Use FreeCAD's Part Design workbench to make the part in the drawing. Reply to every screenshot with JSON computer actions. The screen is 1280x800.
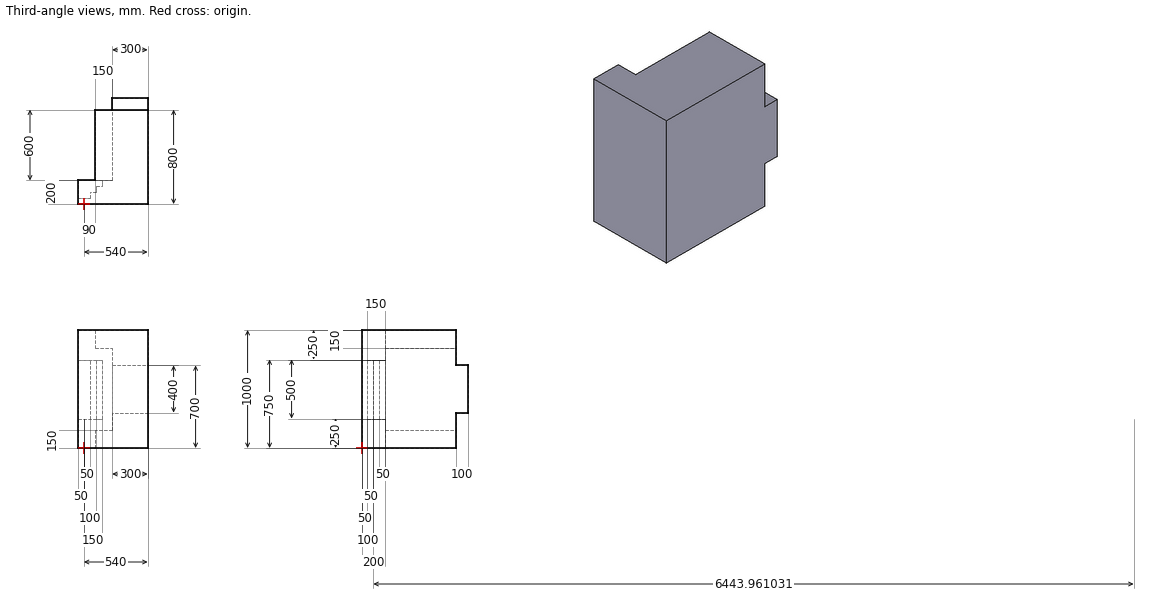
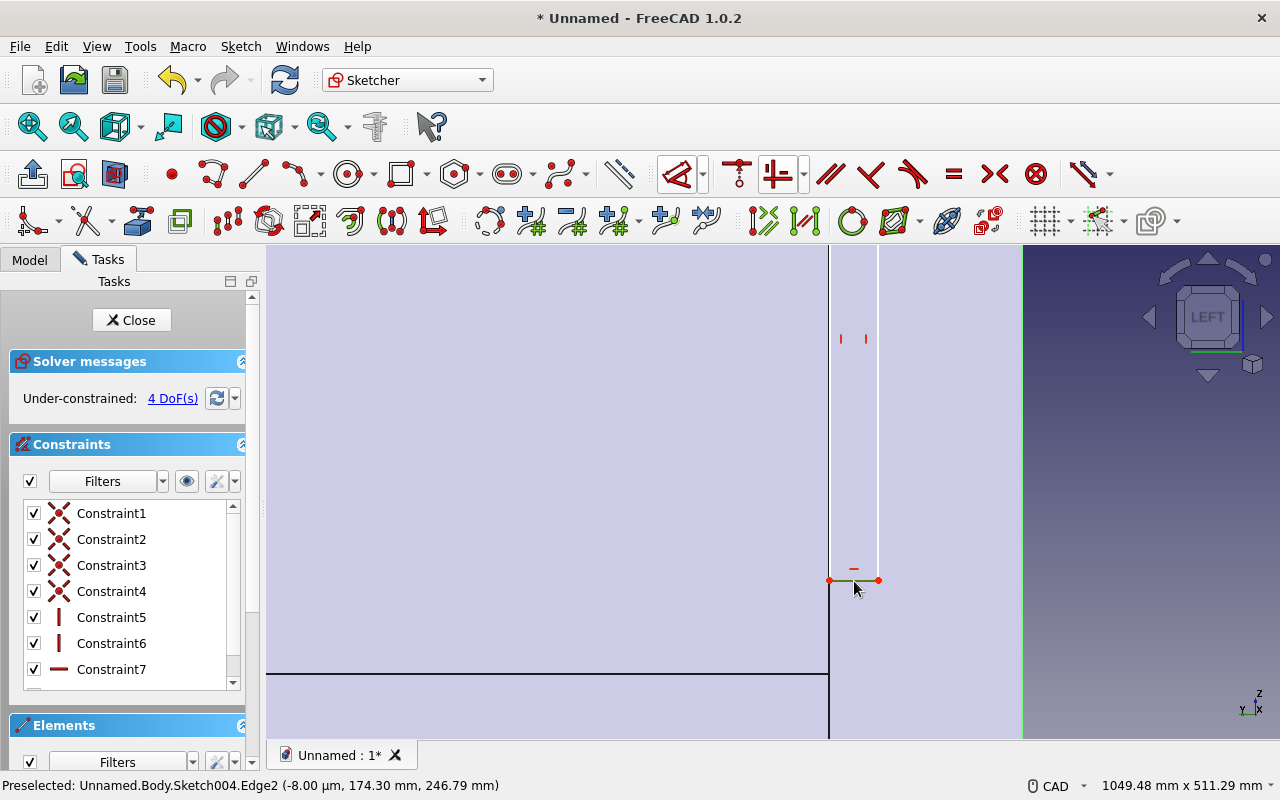
{"action": "key", "text": "l"}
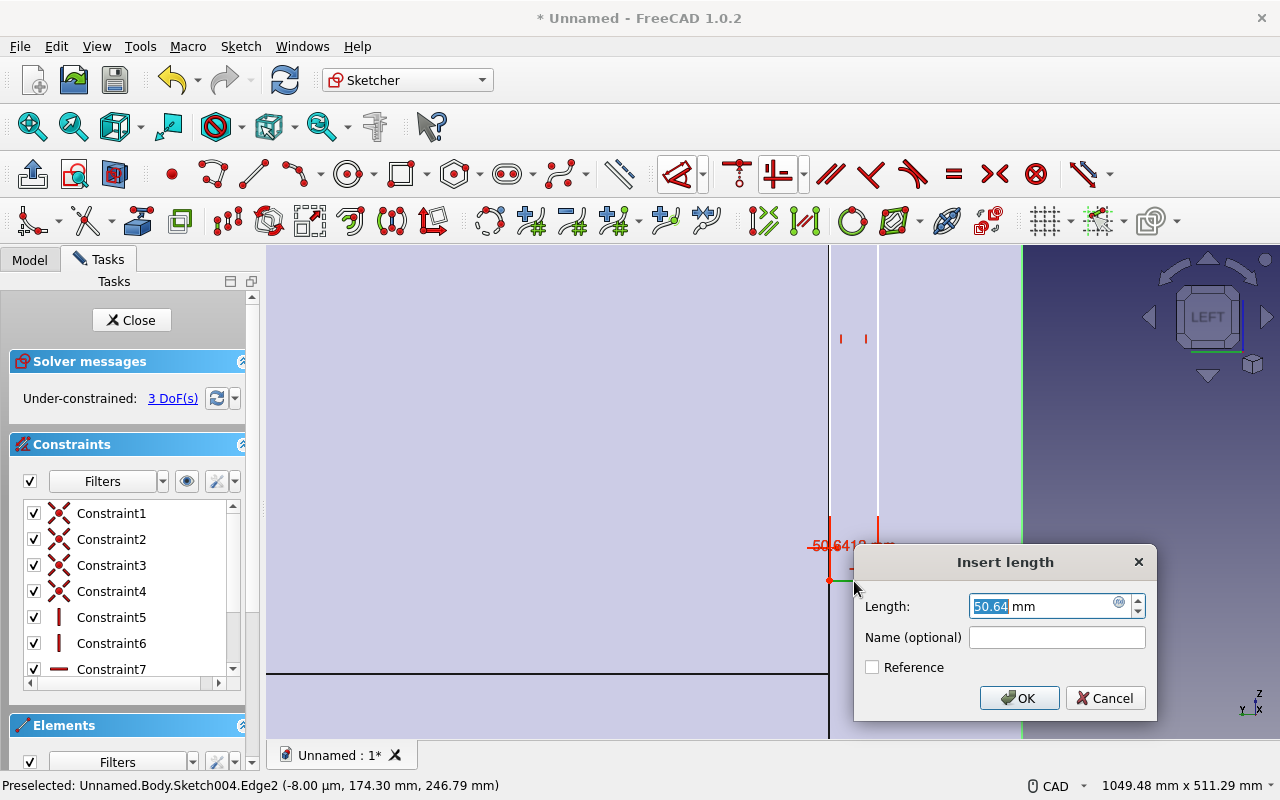
{"action": "type", "text": "50"}
{"action": "key", "text": "Return"}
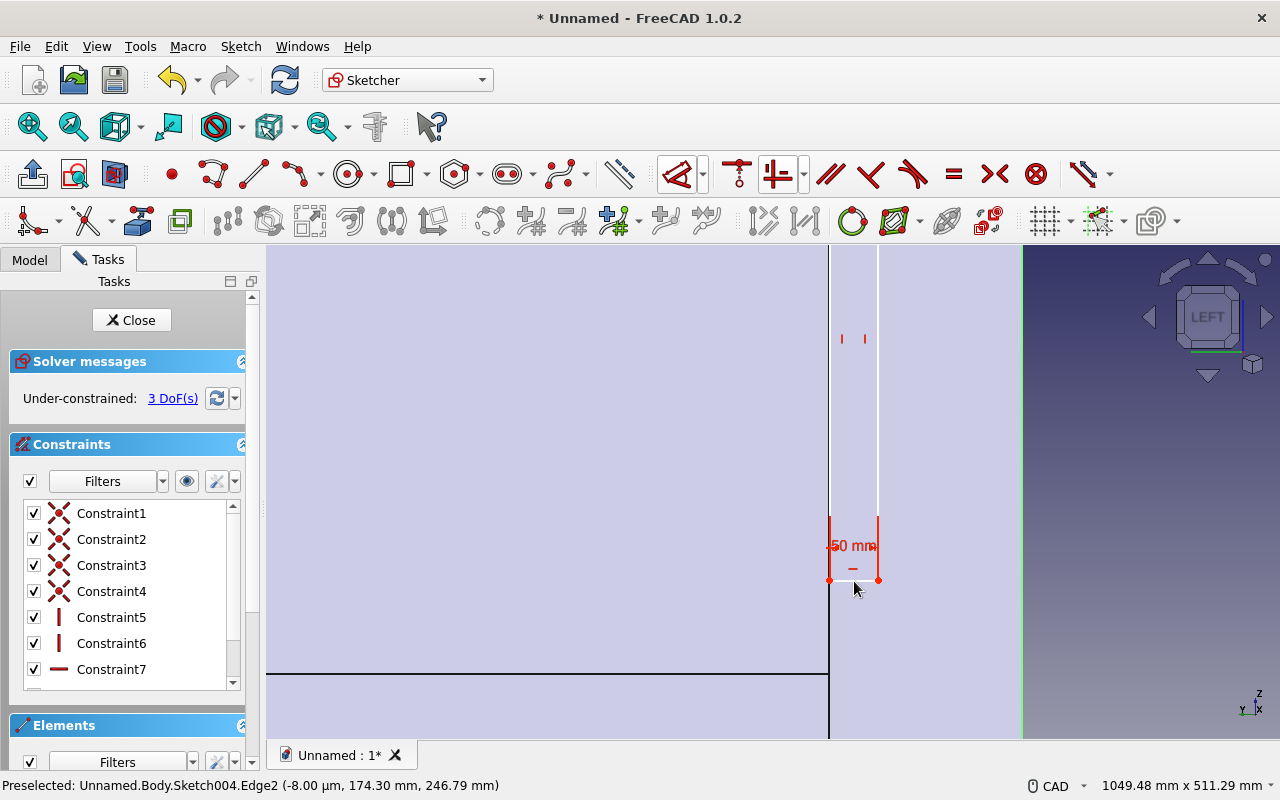
{"action": "left_click", "coordinate": [830, 436]}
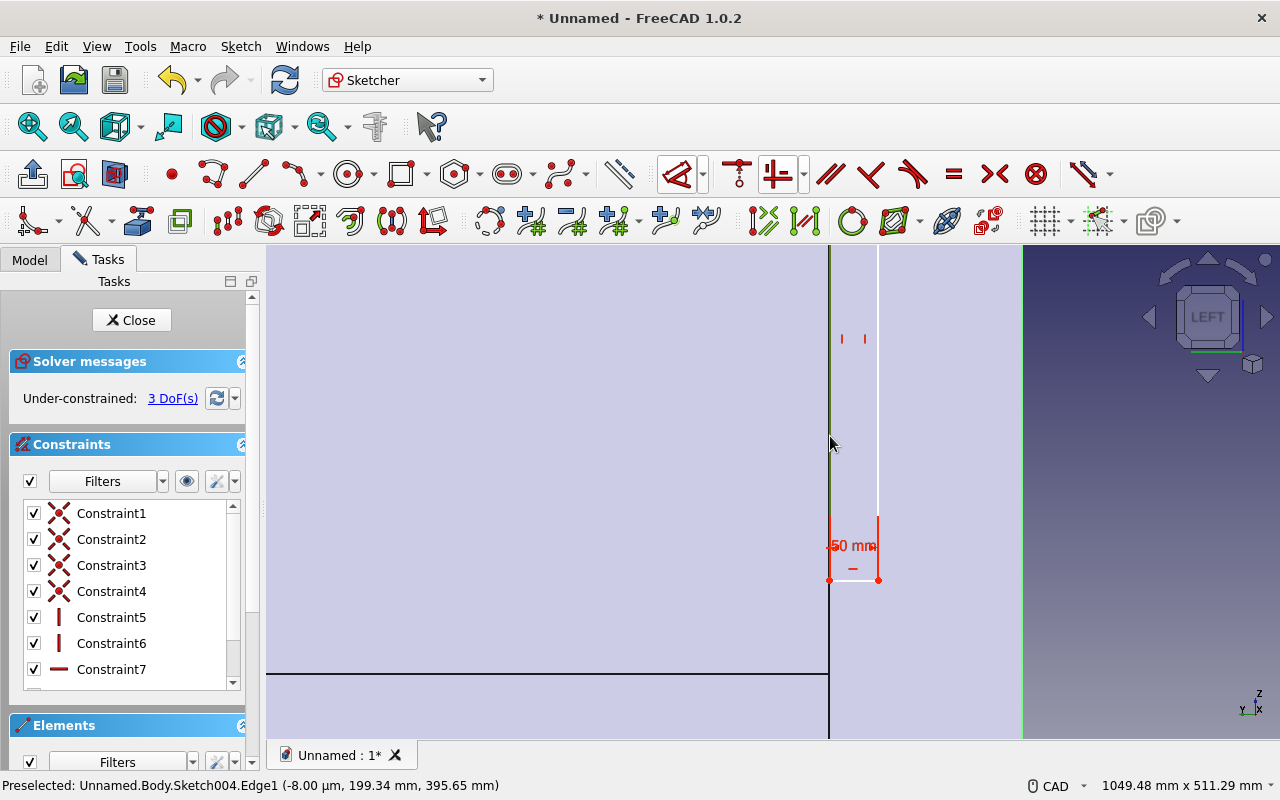
{"action": "left_click", "coordinate": [702, 174]}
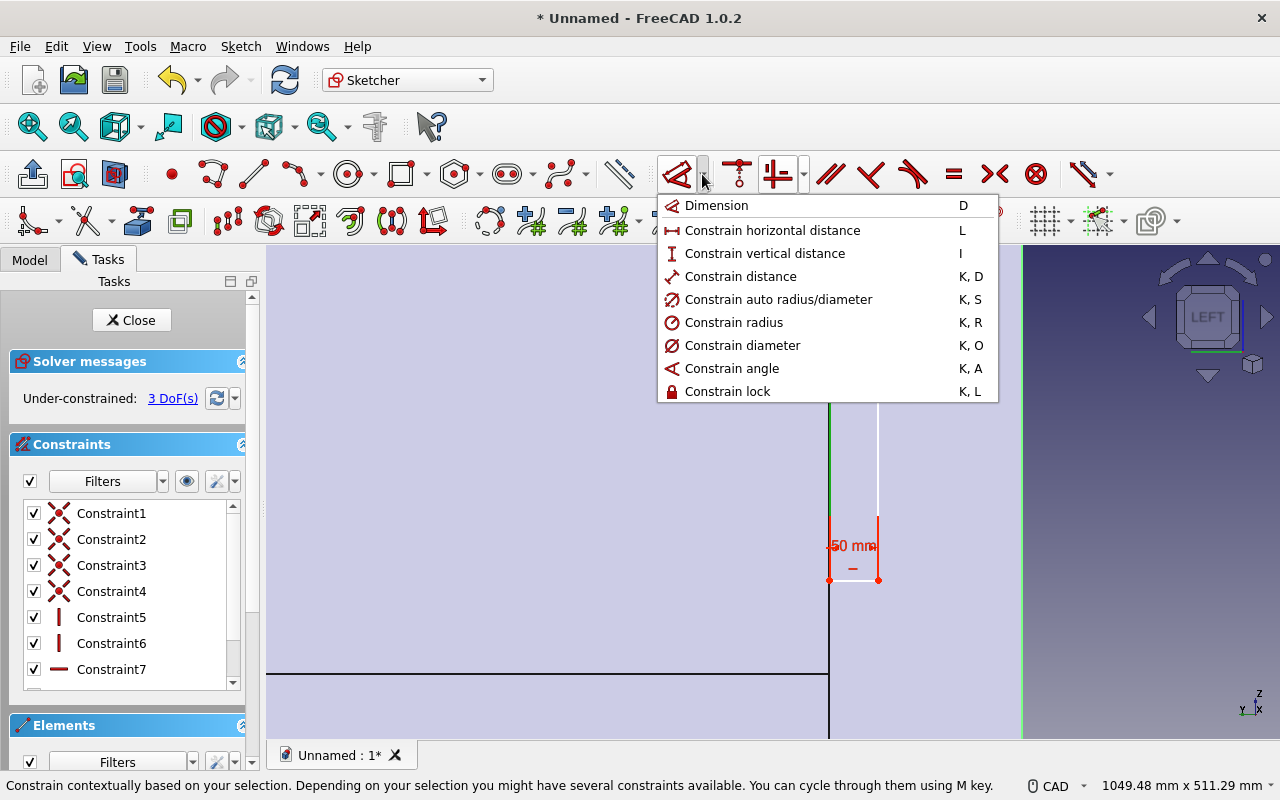
{"action": "left_click", "coordinate": [828, 254]}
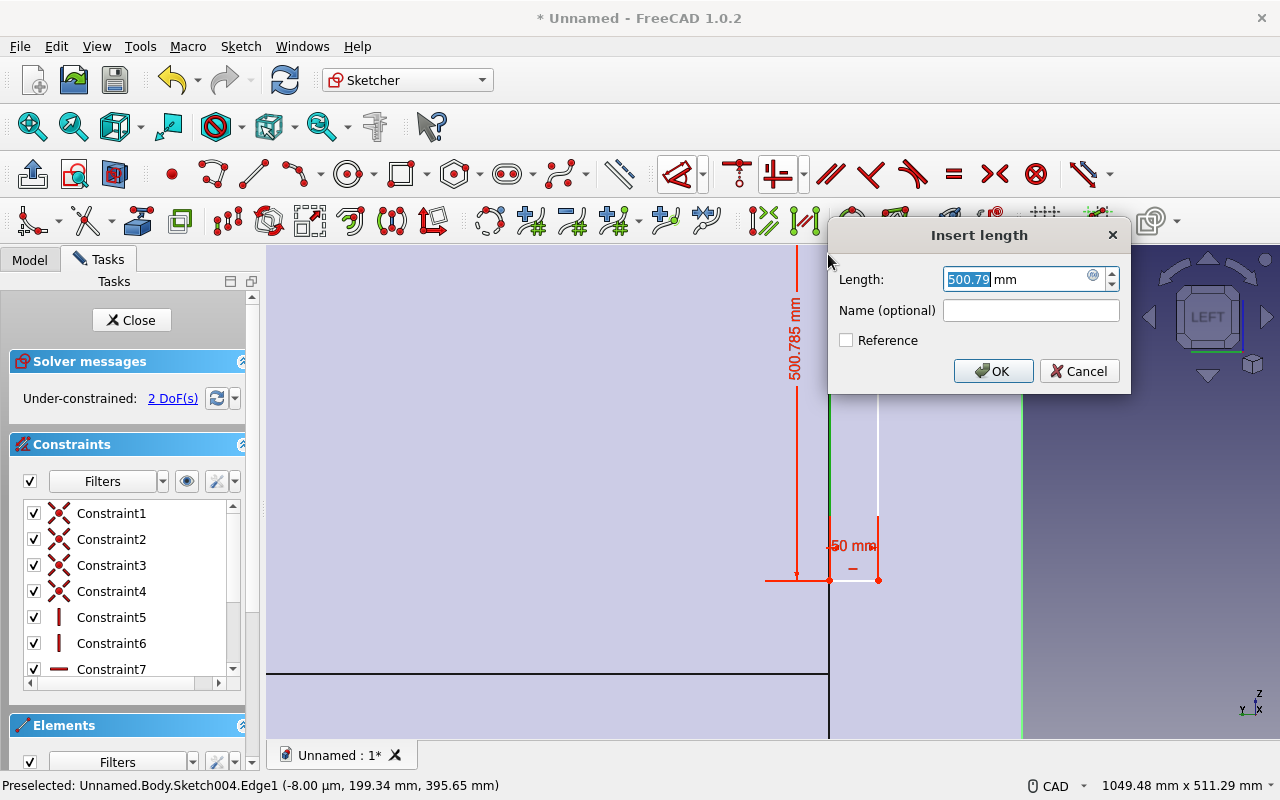
{"action": "type", "text": "500"}
{"action": "key", "text": "Return"}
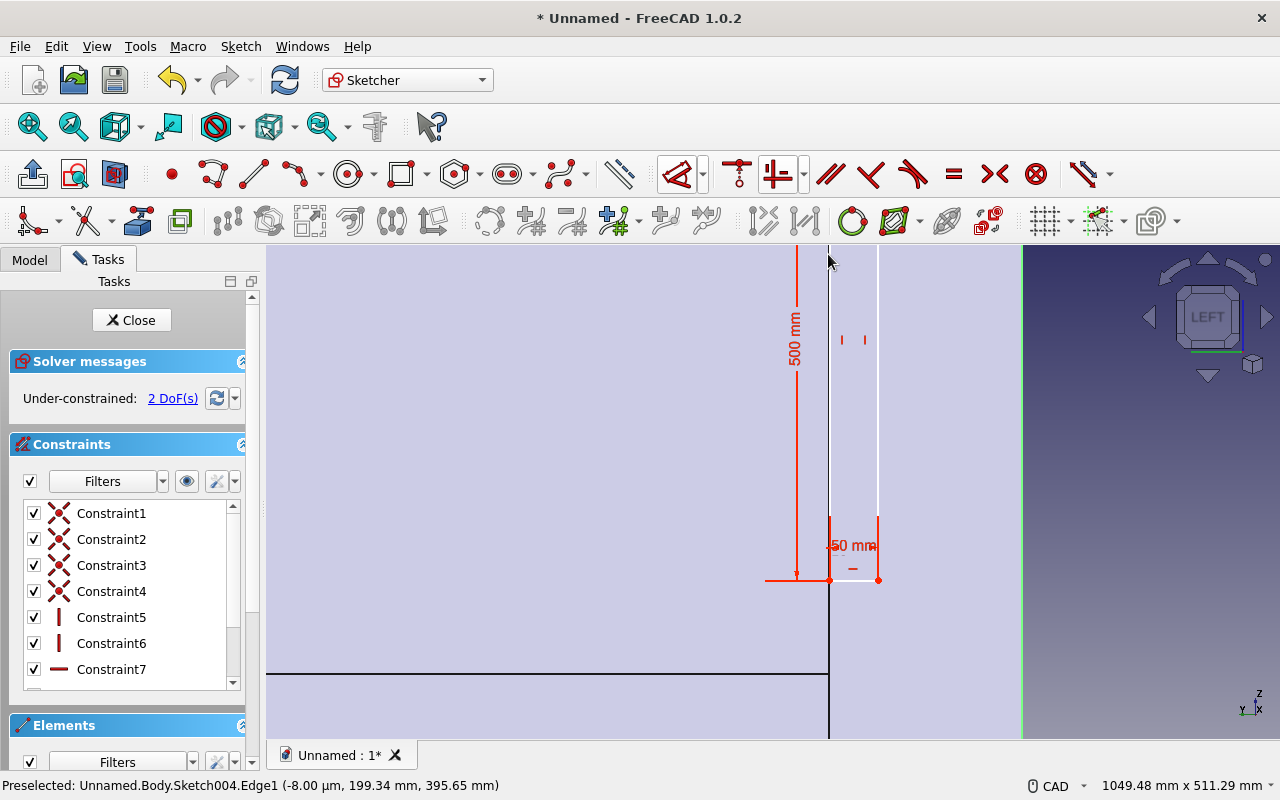
{"action": "scroll", "coordinate": [524, 521], "scroll_direction": "down", "scroll_amount": 4}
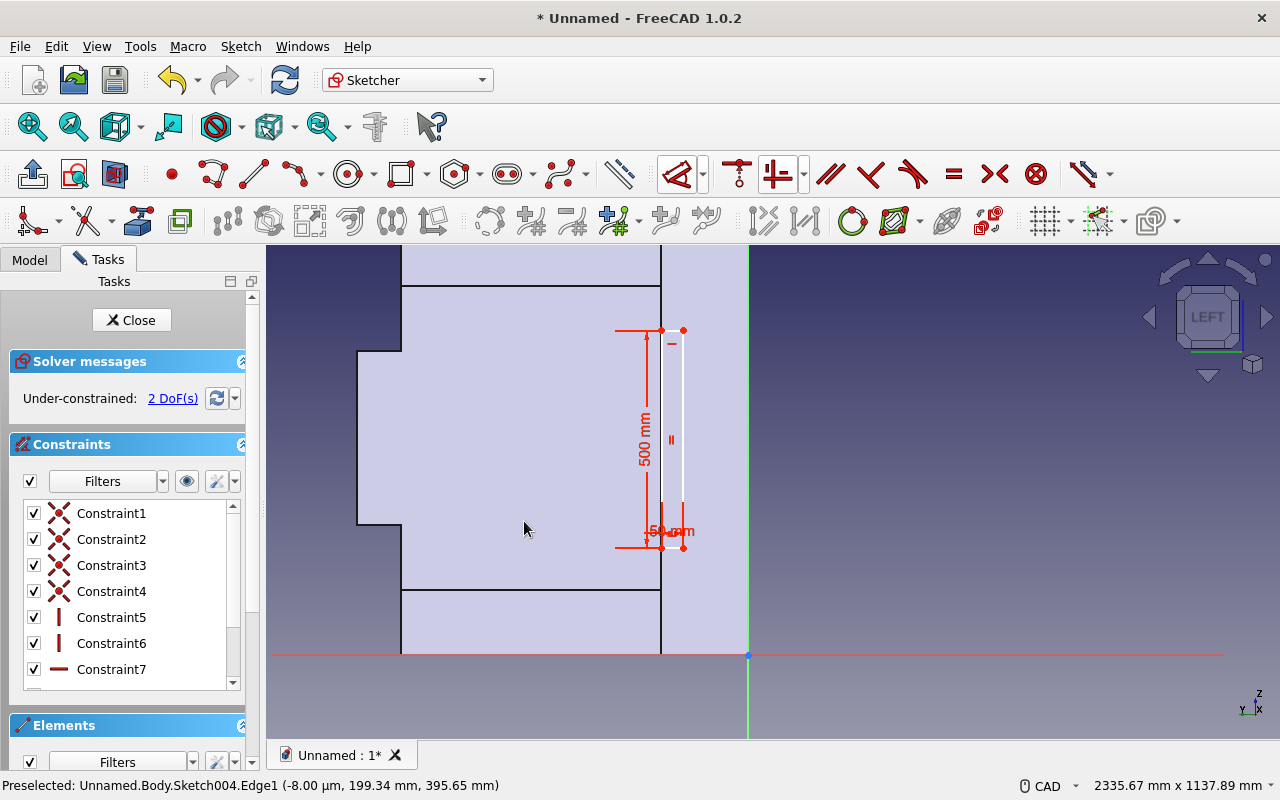
{"action": "left_click", "coordinate": [662, 331]}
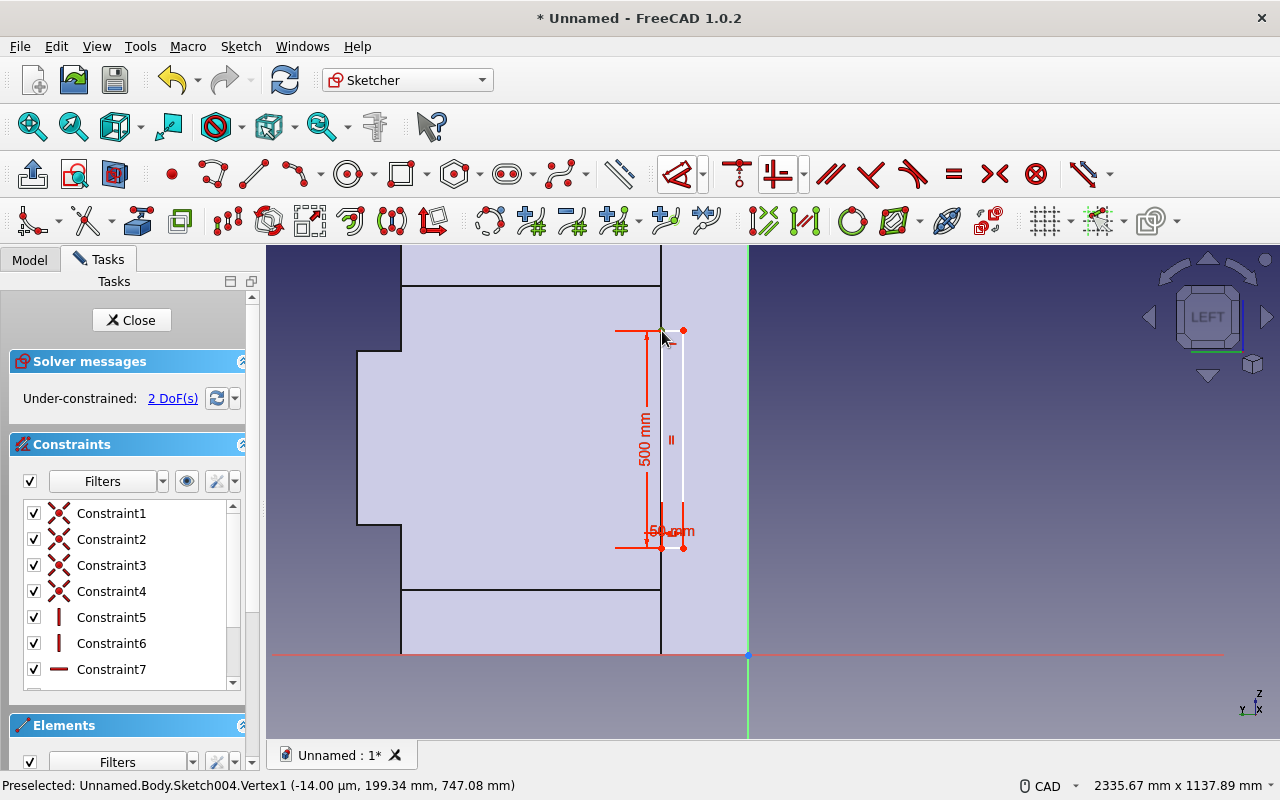
{"action": "key", "text": "l"}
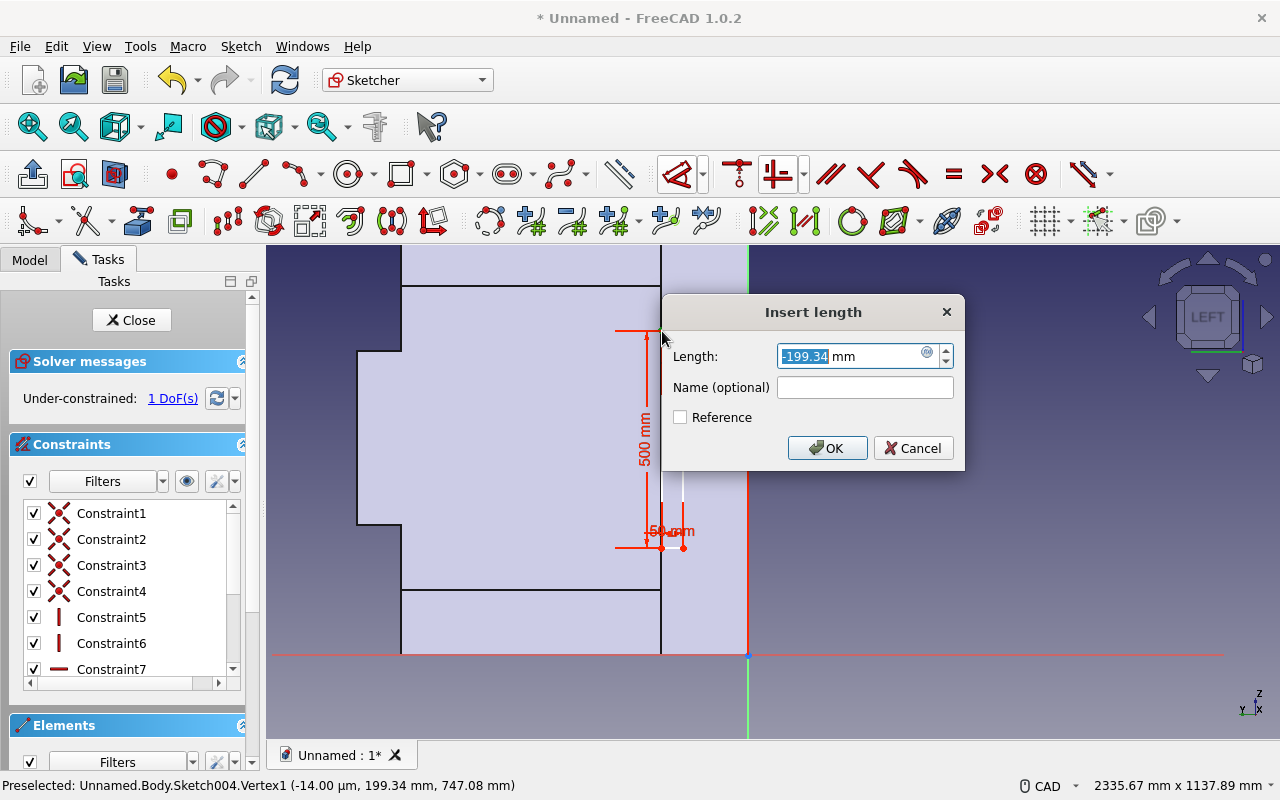
{"action": "type", "text": "-200"}
{"action": "key", "text": "Return"}